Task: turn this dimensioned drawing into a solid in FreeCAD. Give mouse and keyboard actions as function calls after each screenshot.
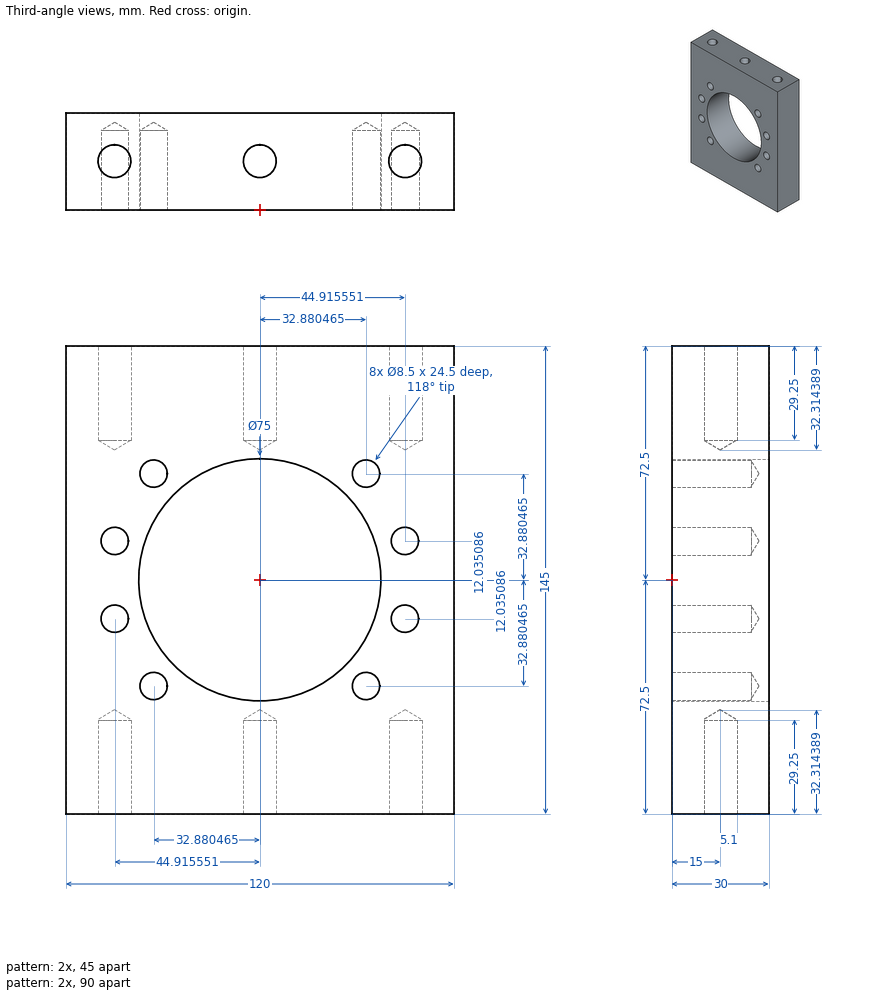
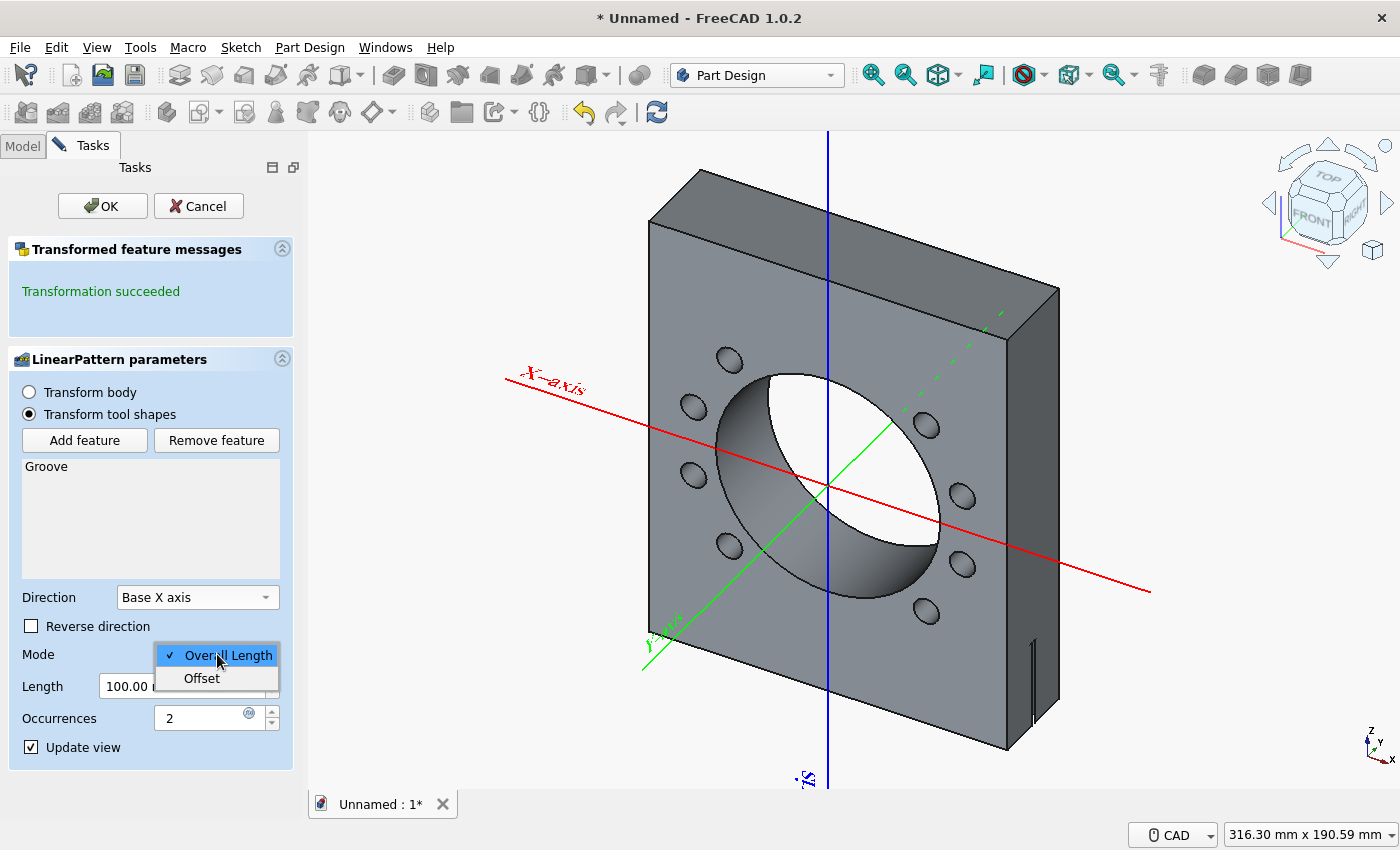
click(216, 678)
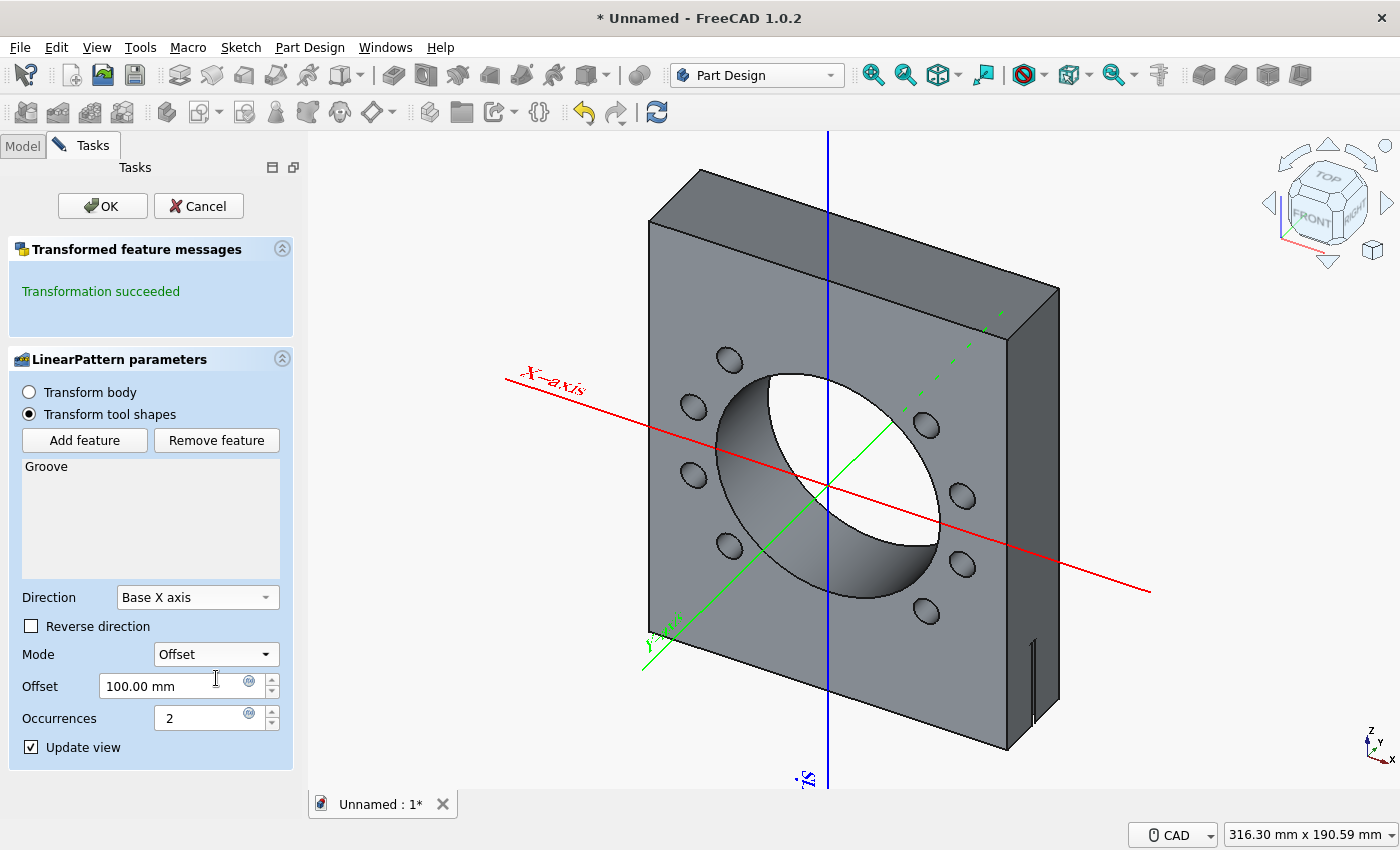
triple_click(182, 686)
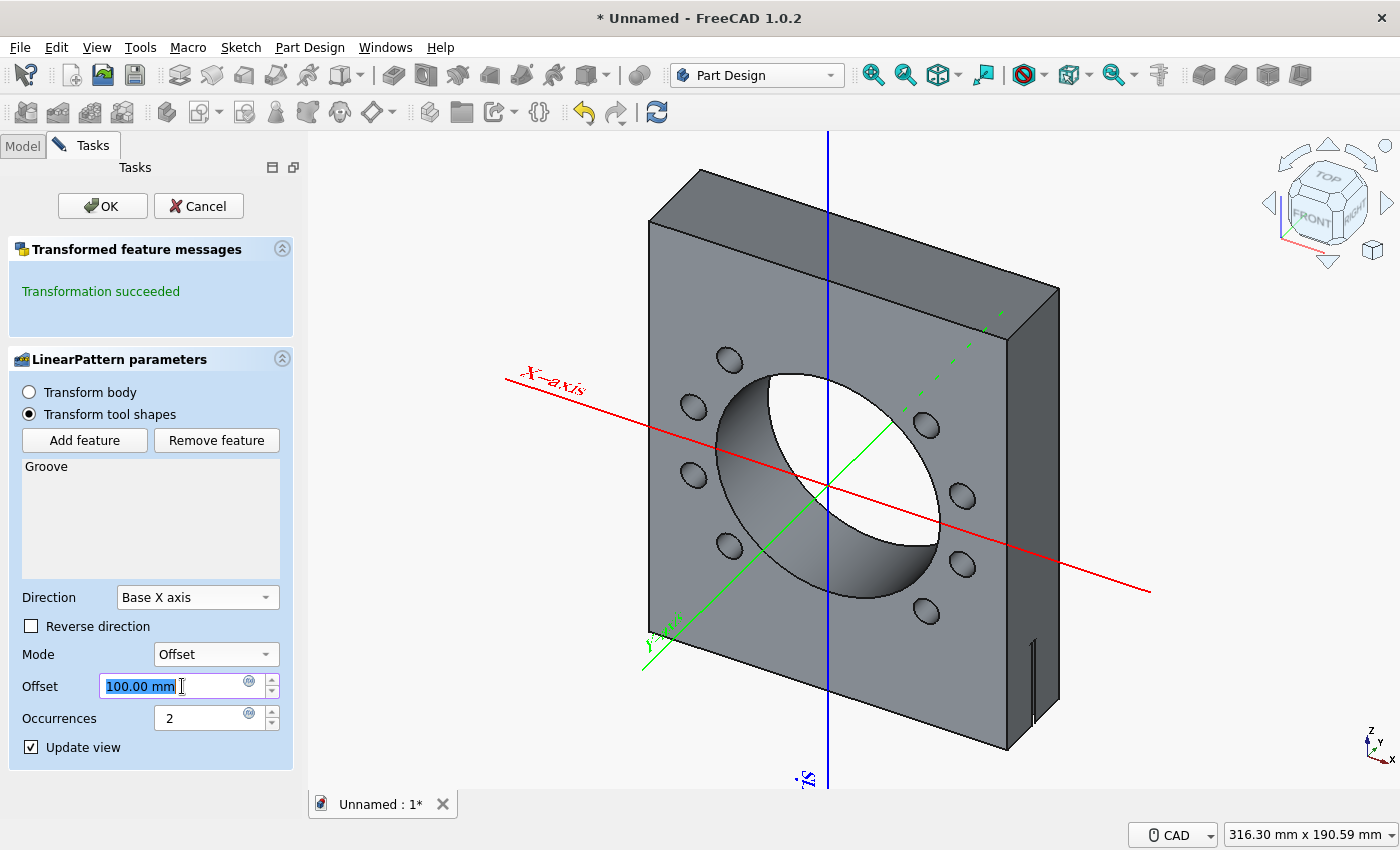
text(45)
key(Tab)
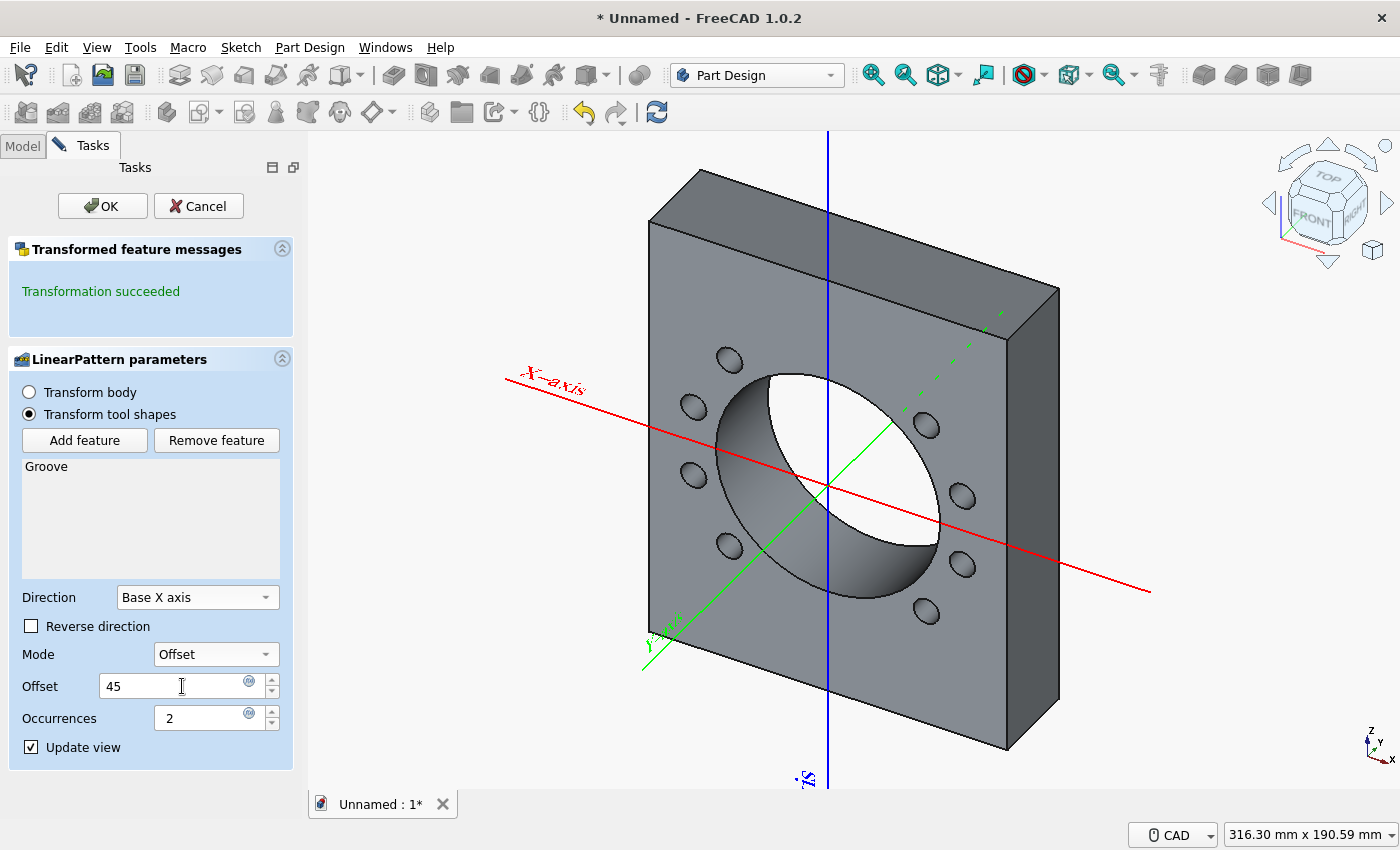
triple_click(209, 718)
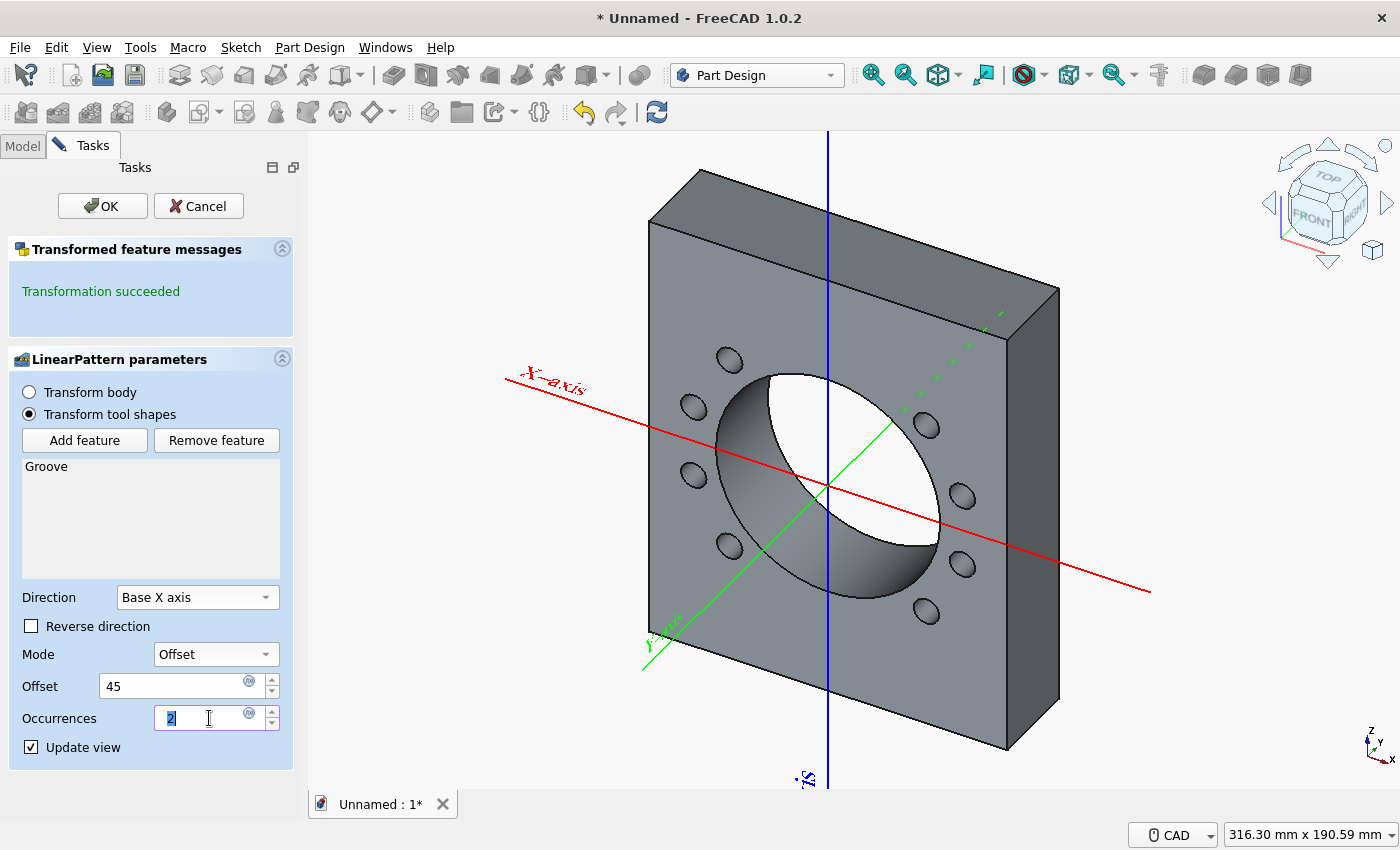
text(2)
key(Tab)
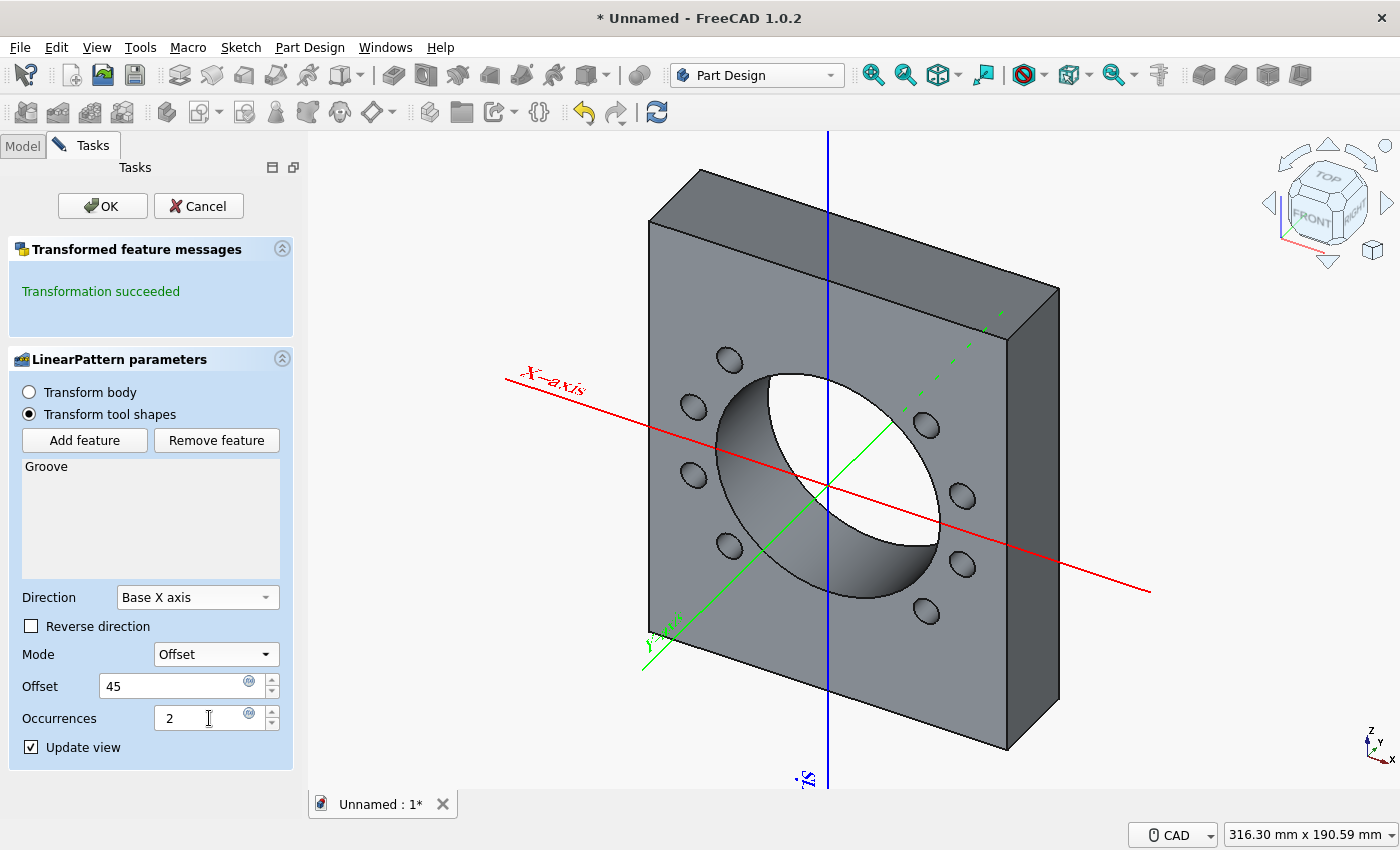
click(103, 206)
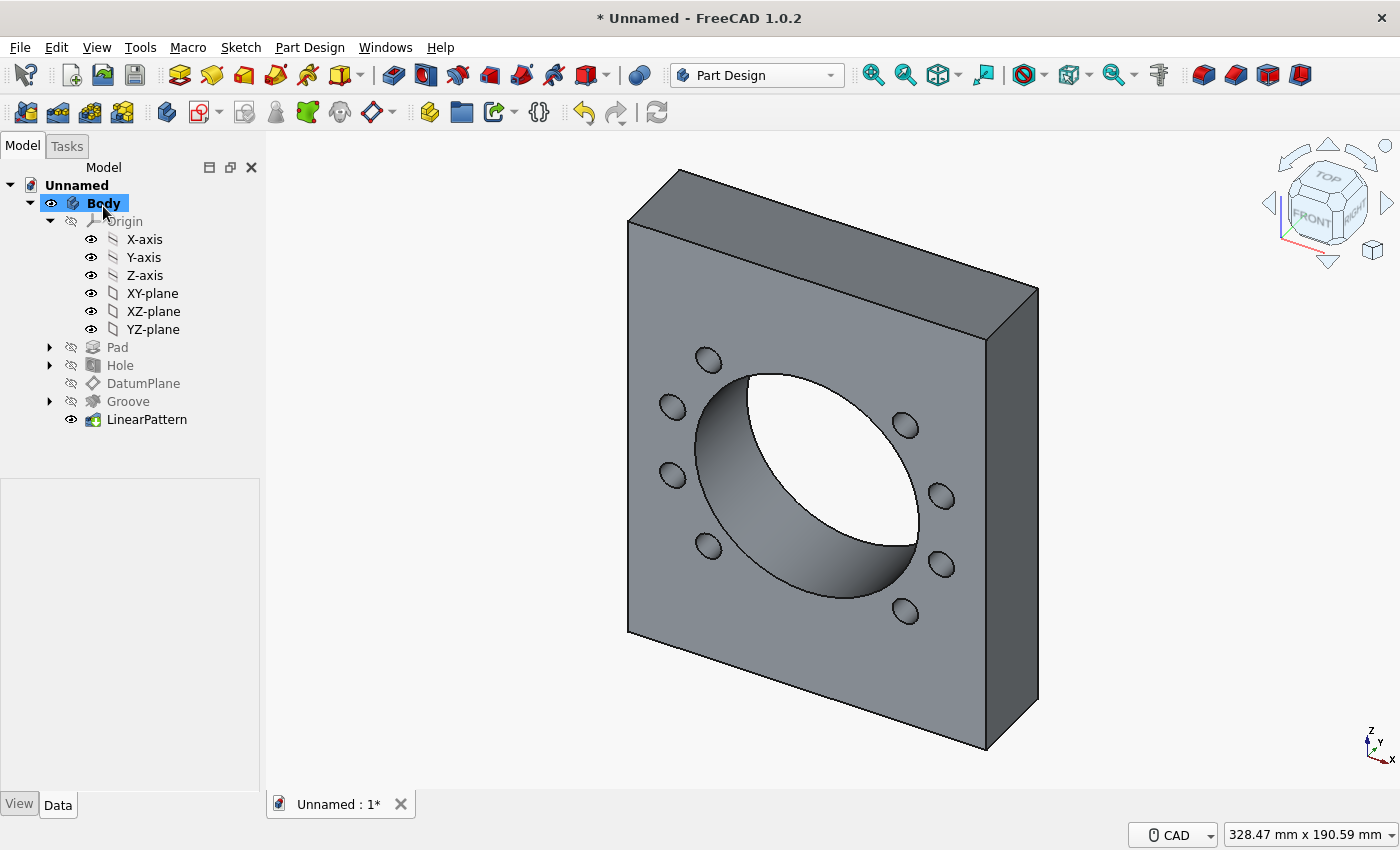
click(116, 401)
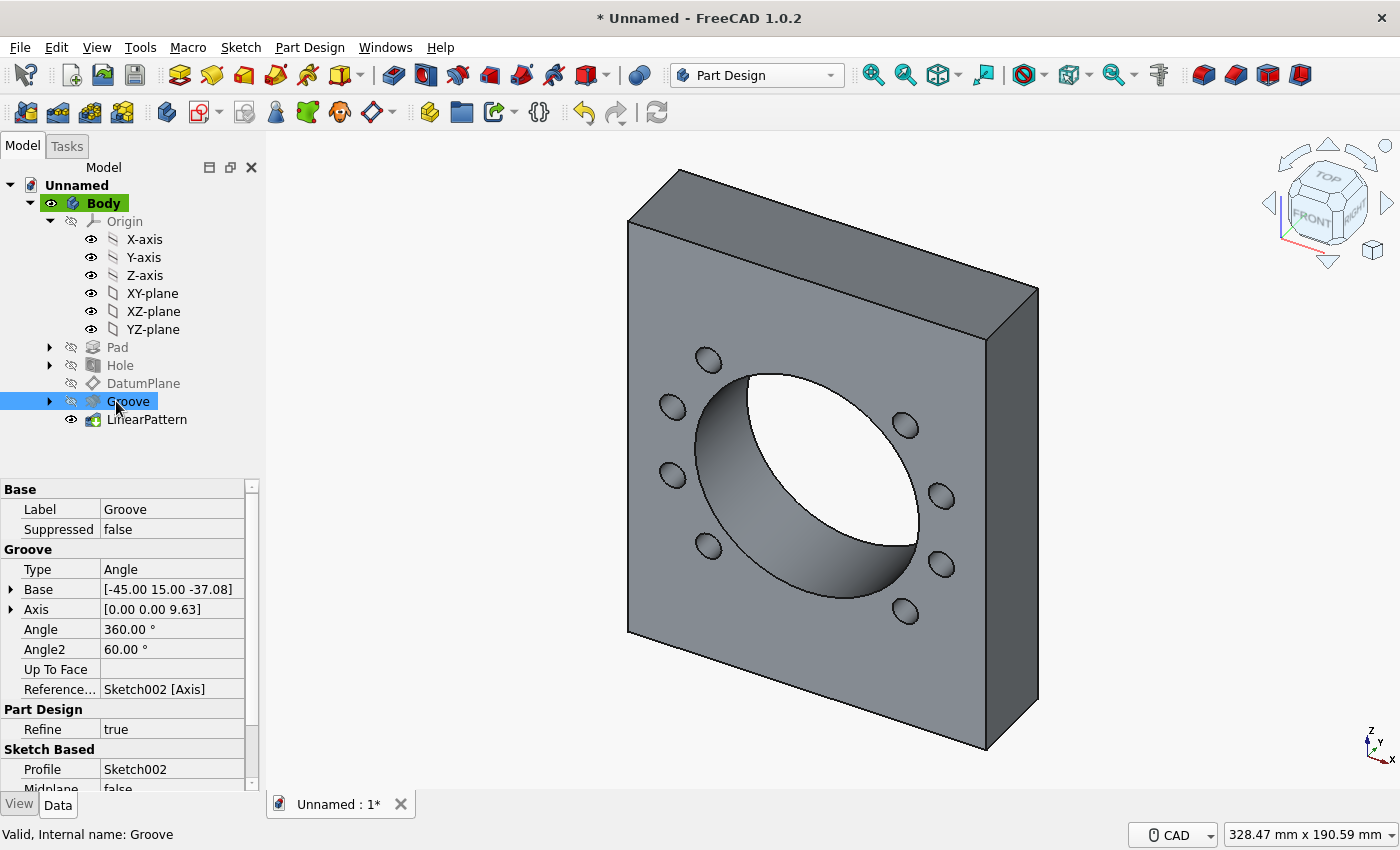
click(58, 112)